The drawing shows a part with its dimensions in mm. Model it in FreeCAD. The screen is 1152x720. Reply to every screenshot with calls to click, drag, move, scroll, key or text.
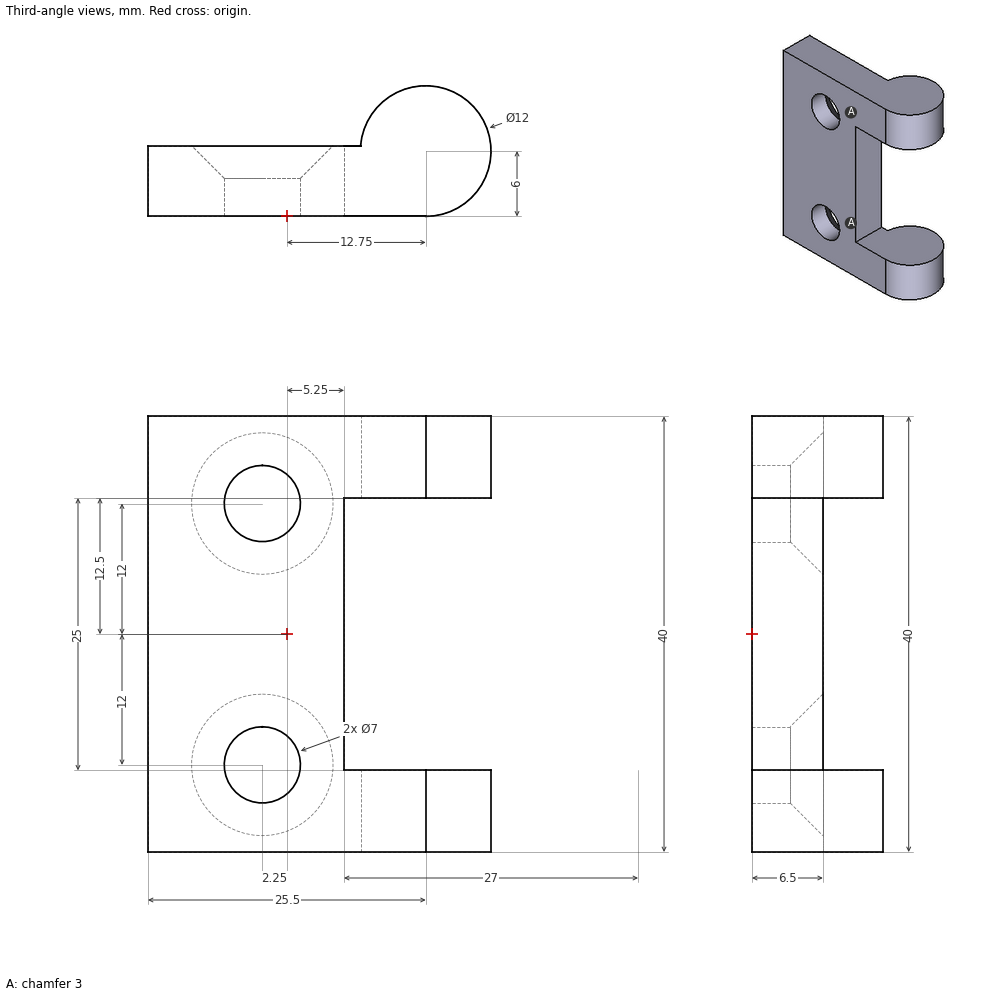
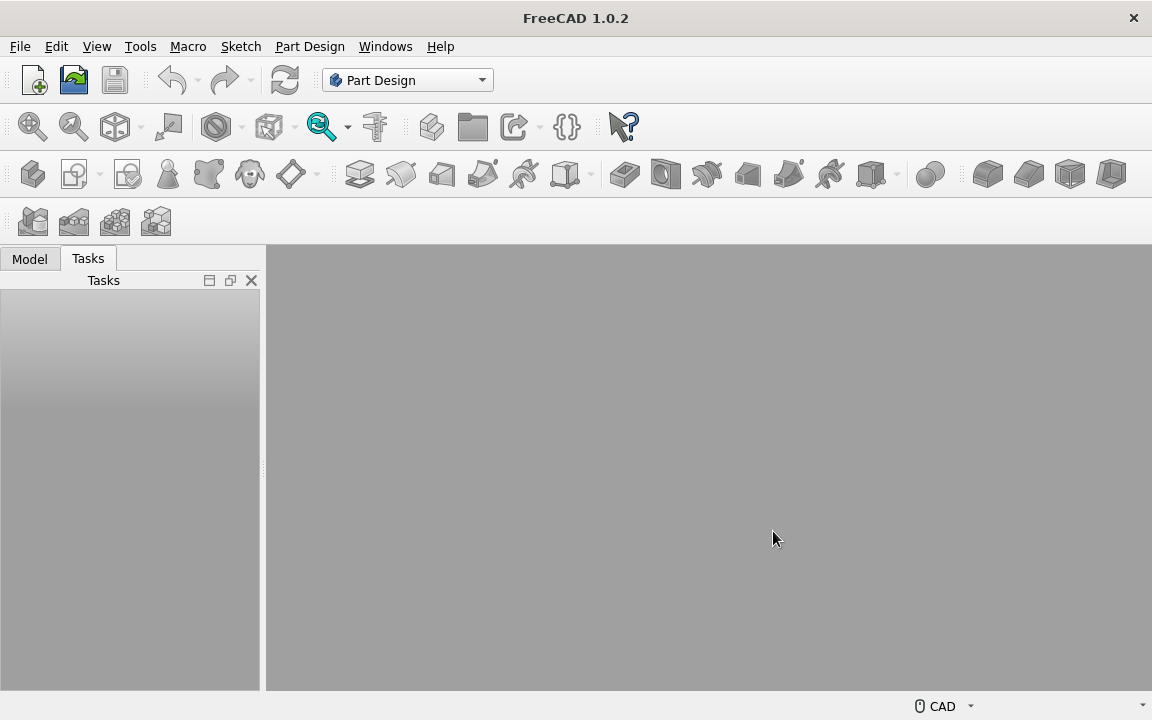
click(33, 80)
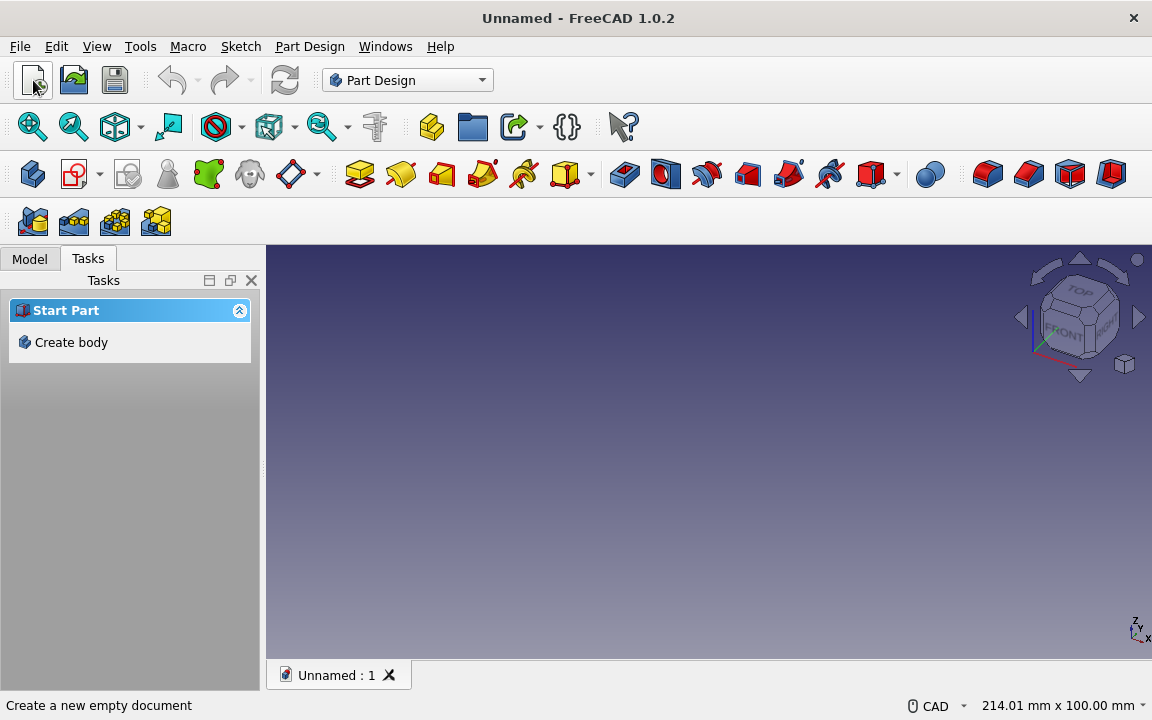
click(74, 174)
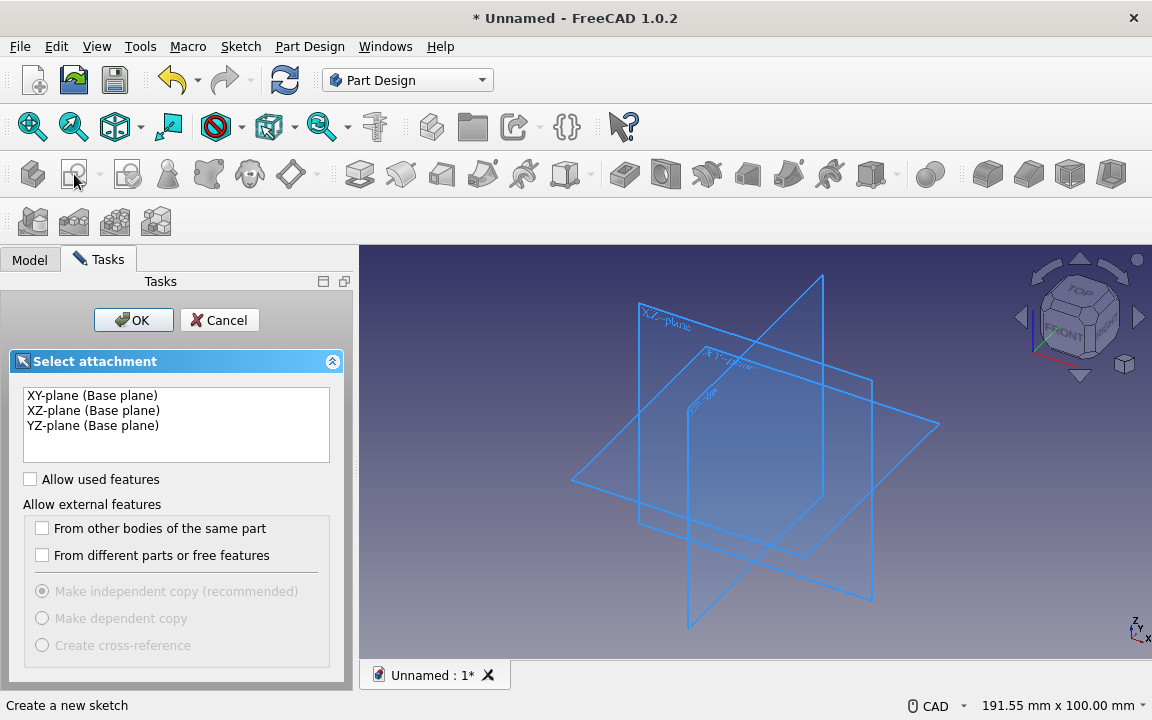
click(84, 410)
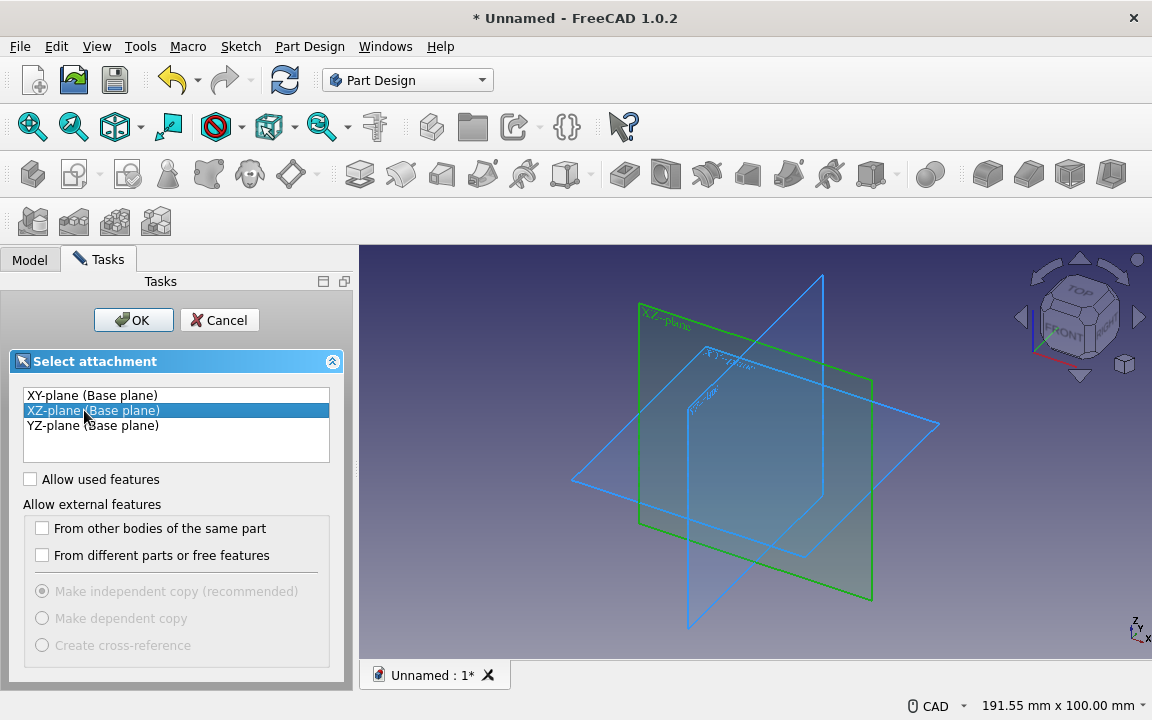
click(134, 320)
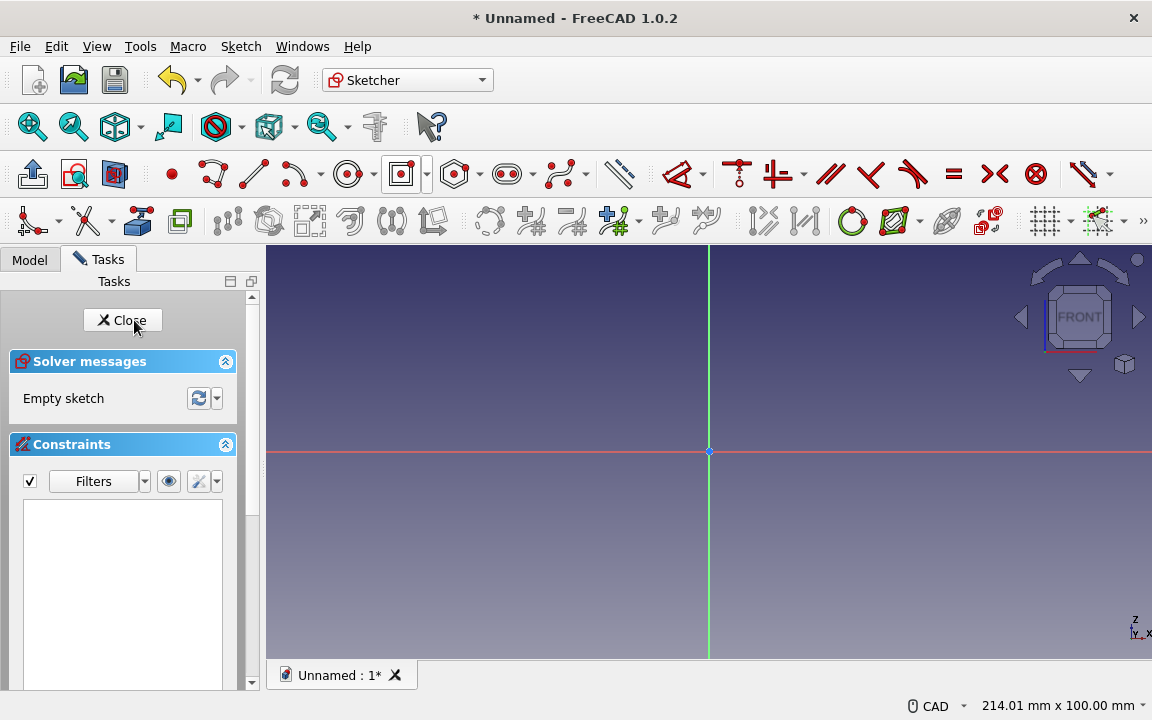
scroll(848, 452, up, 2)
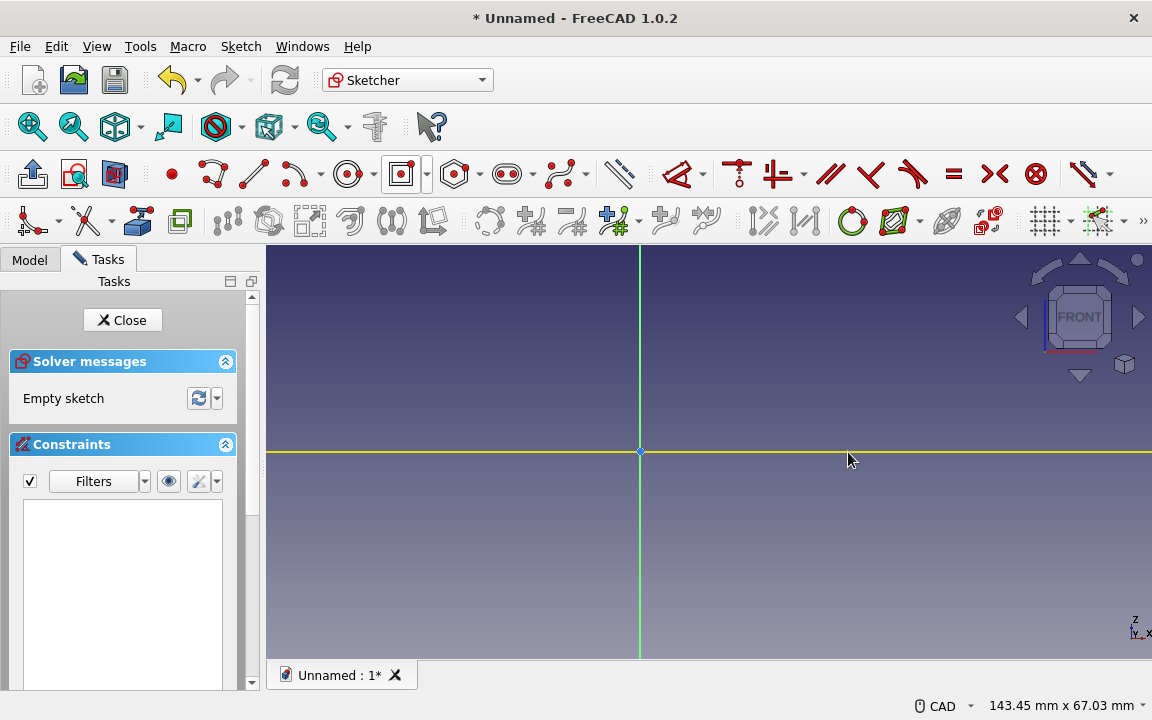
click(400, 174)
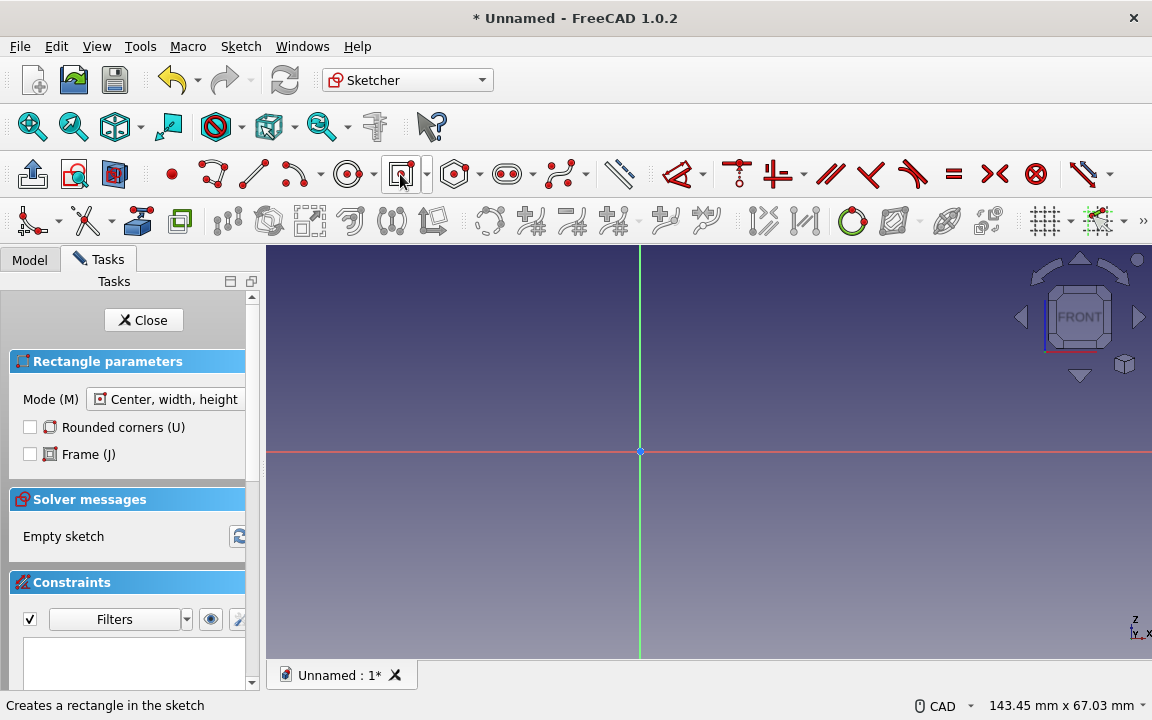
click(640, 452)
click(719, 328)
key(Escape)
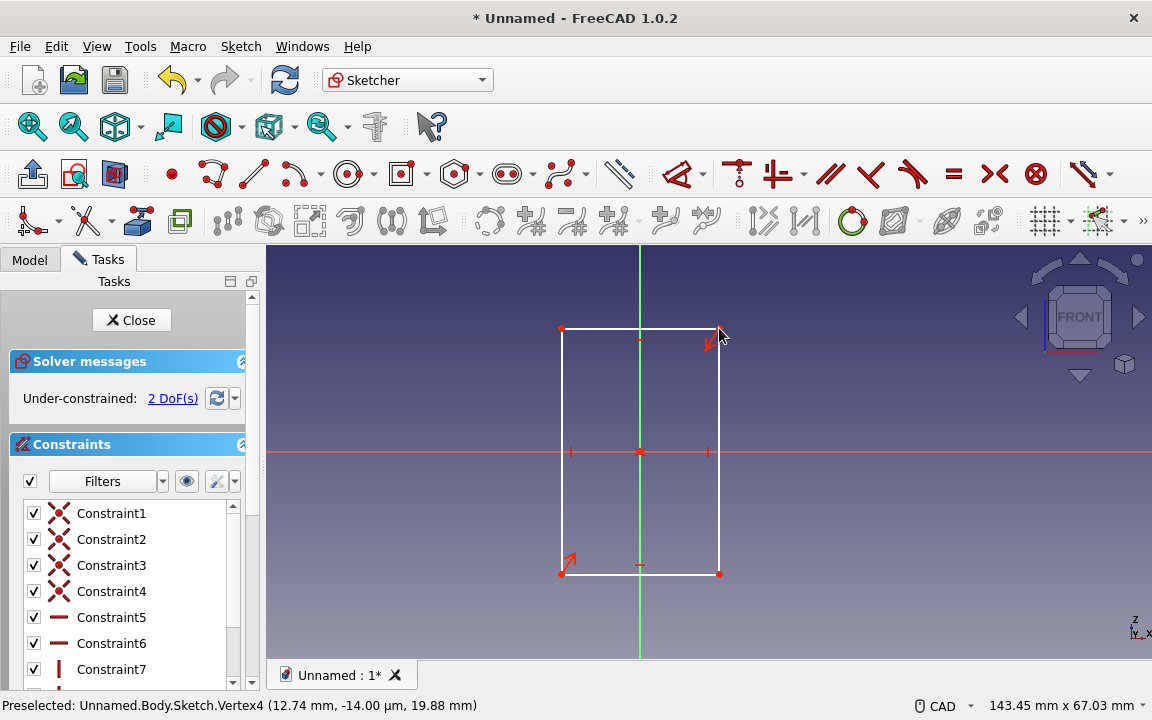
click(676, 174)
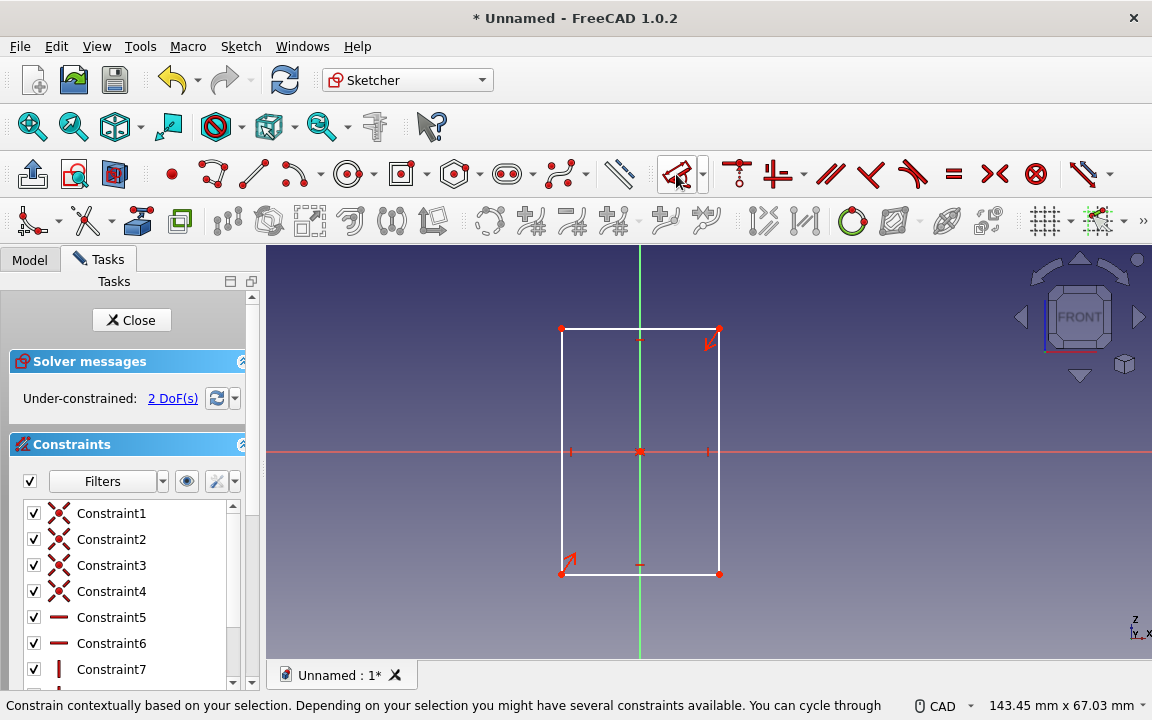
click(719, 501)
click(753, 395)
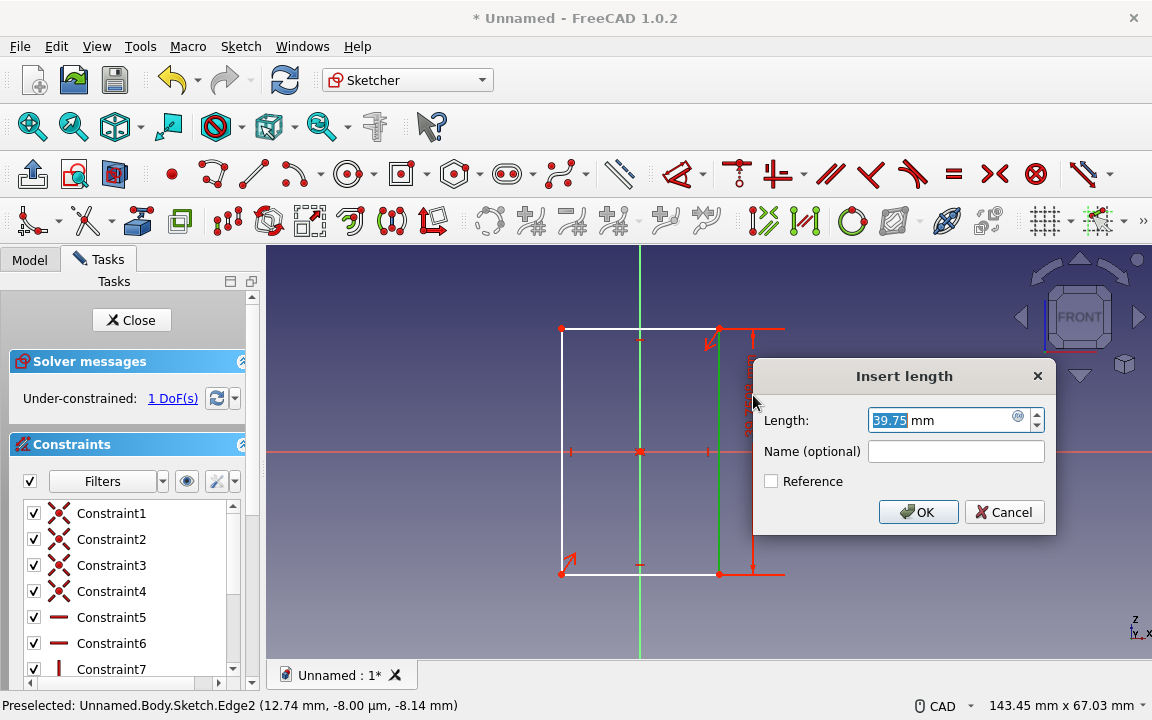
text(40)
key(Return)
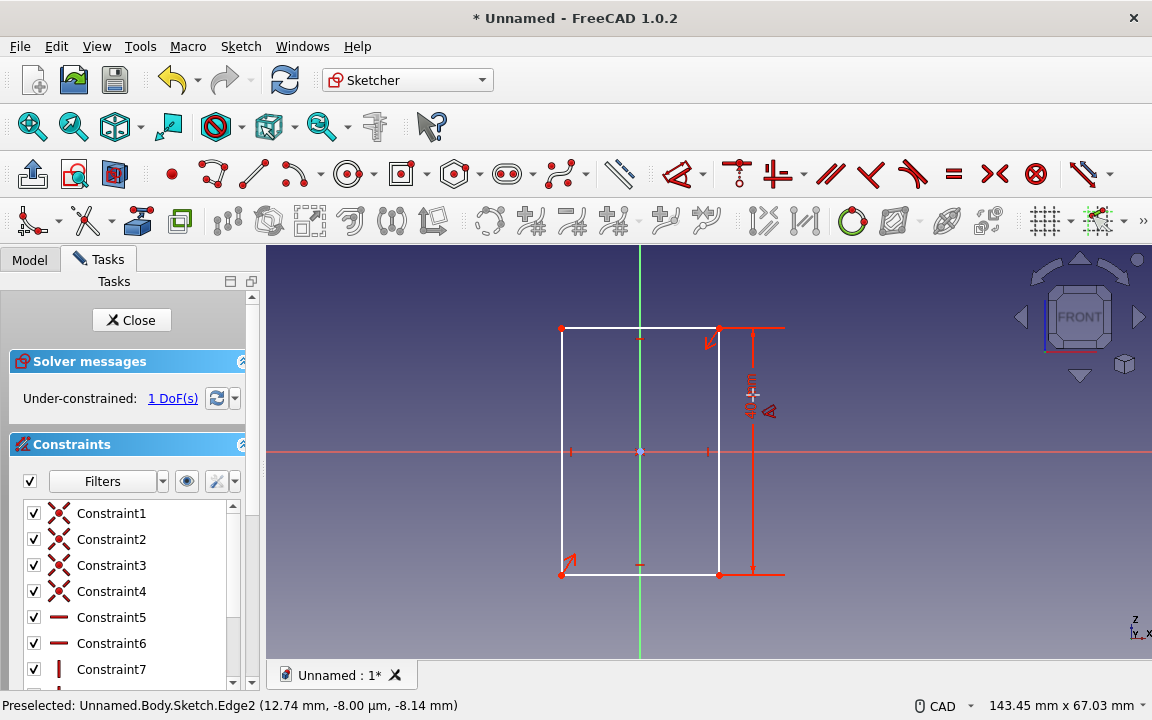
click(609, 575)
click(604, 609)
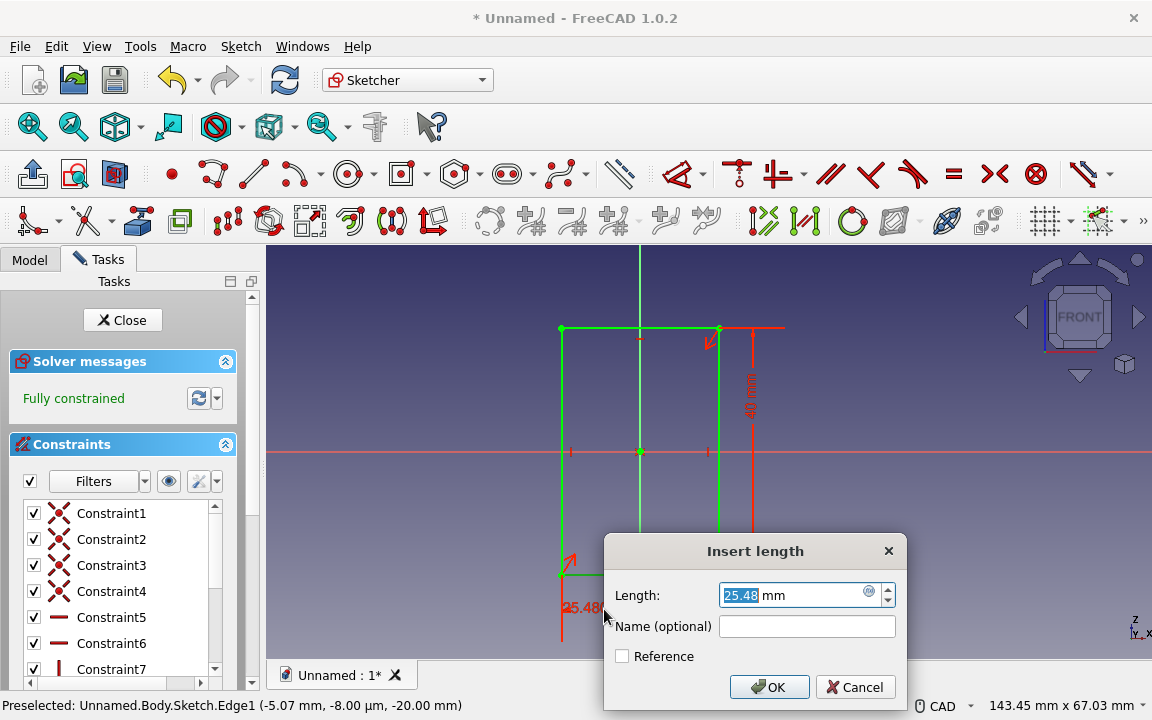
text(25.5)
key(Return)
key(Escape)